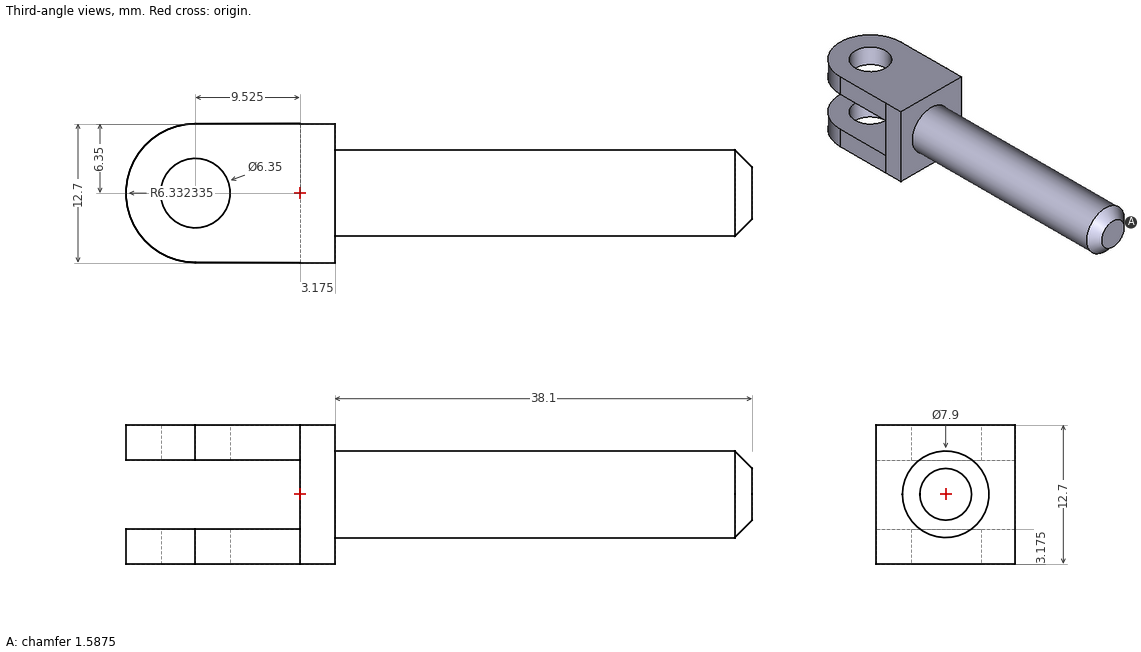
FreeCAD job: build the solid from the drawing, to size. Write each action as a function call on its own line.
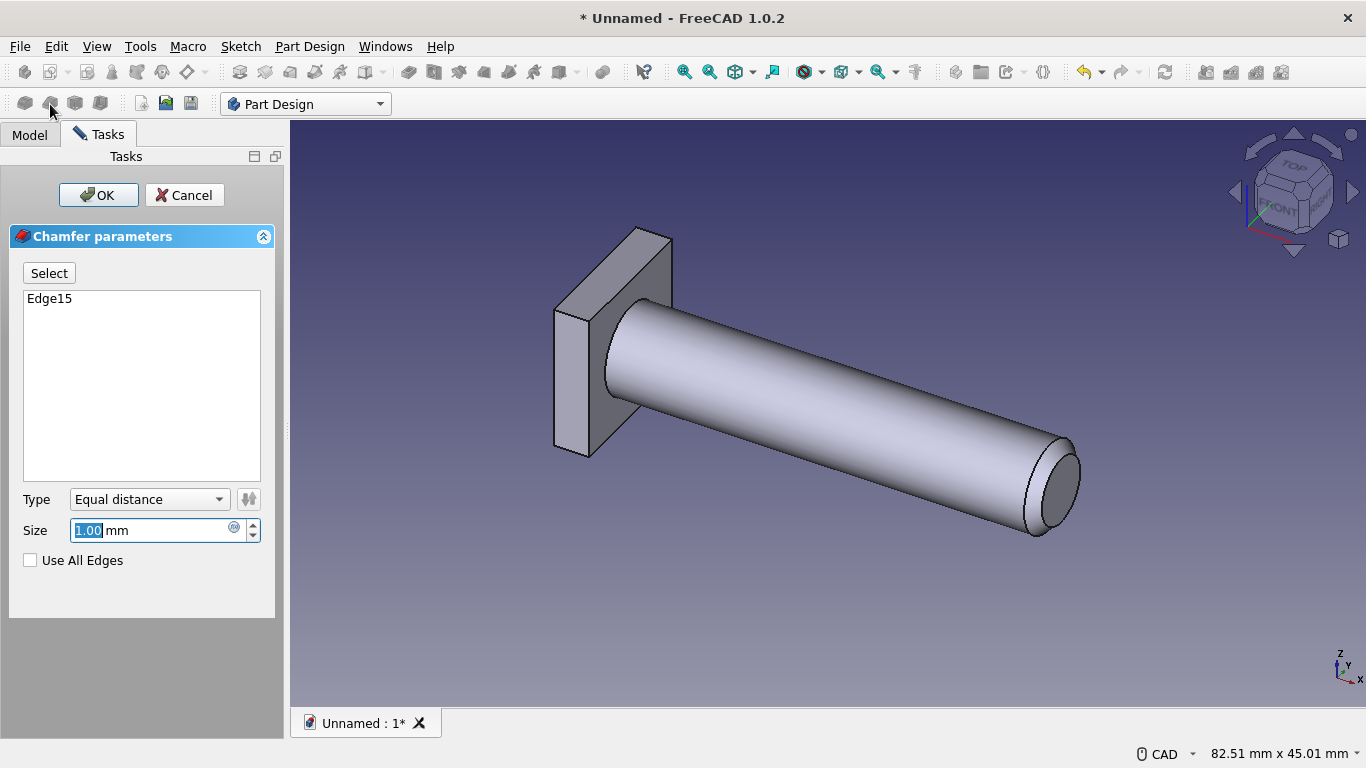
text(1.5875)
key(Tab)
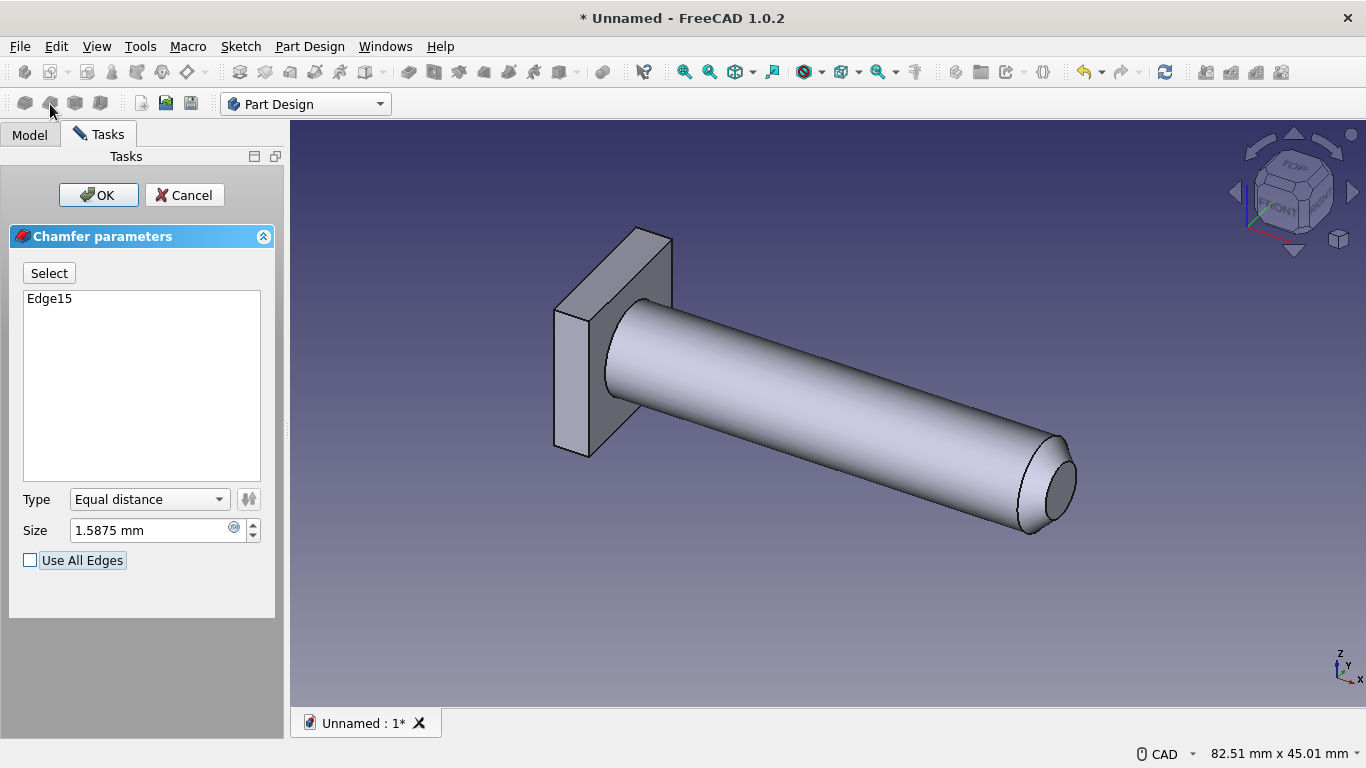
click(99, 195)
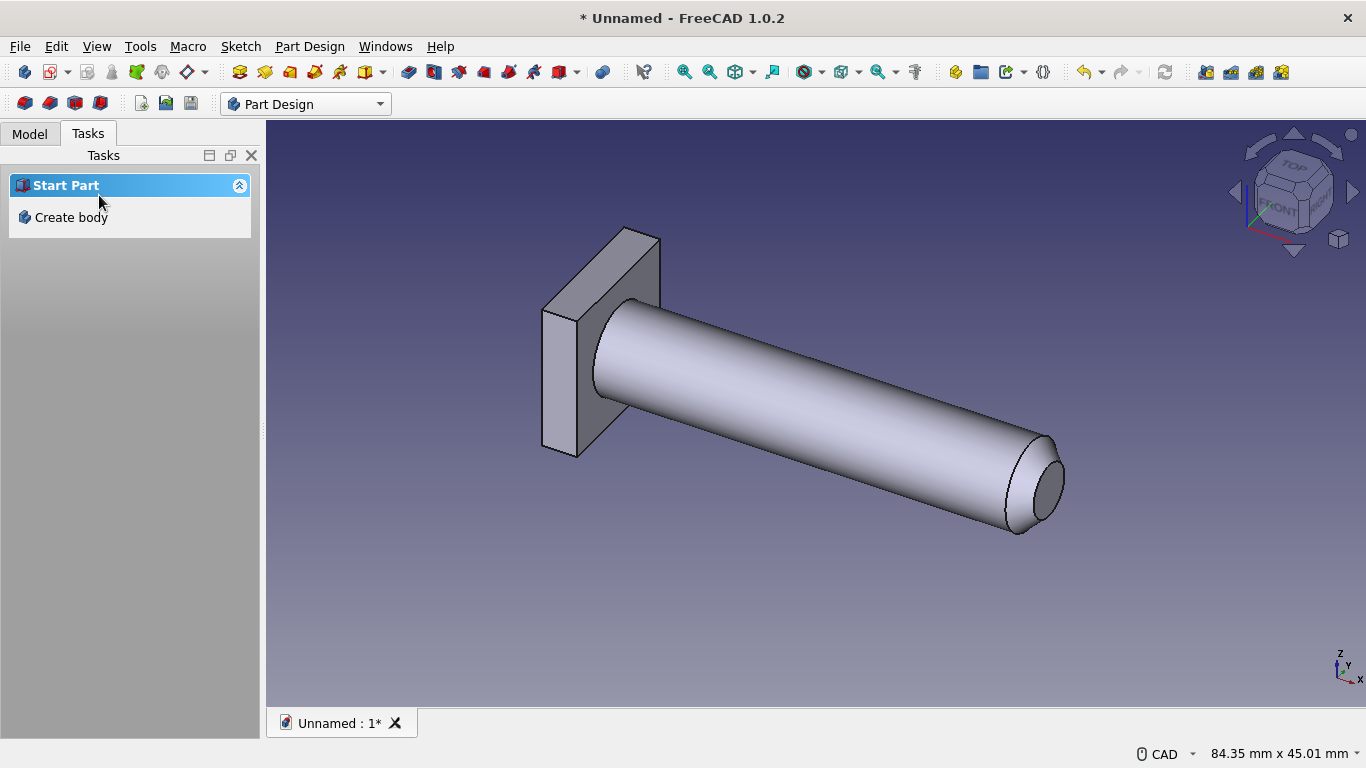
key(5)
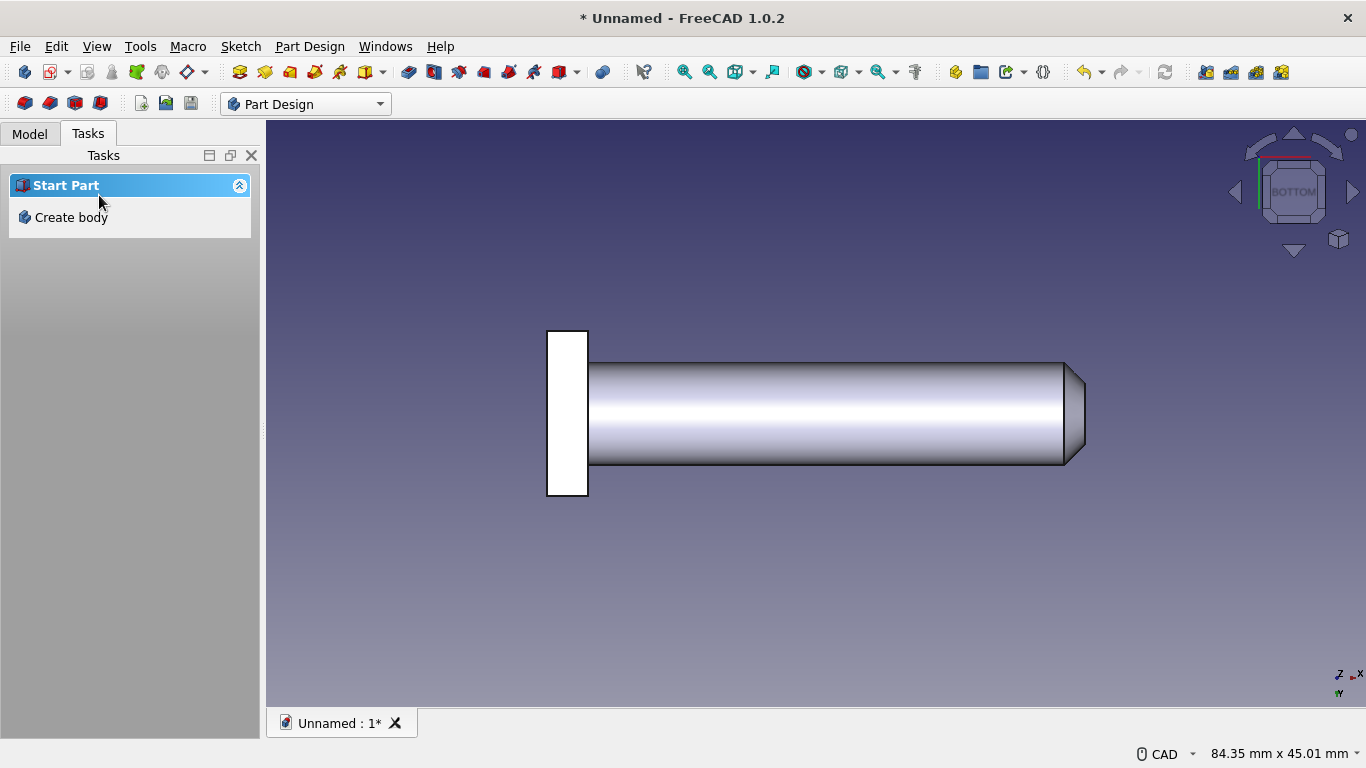
click(568, 460)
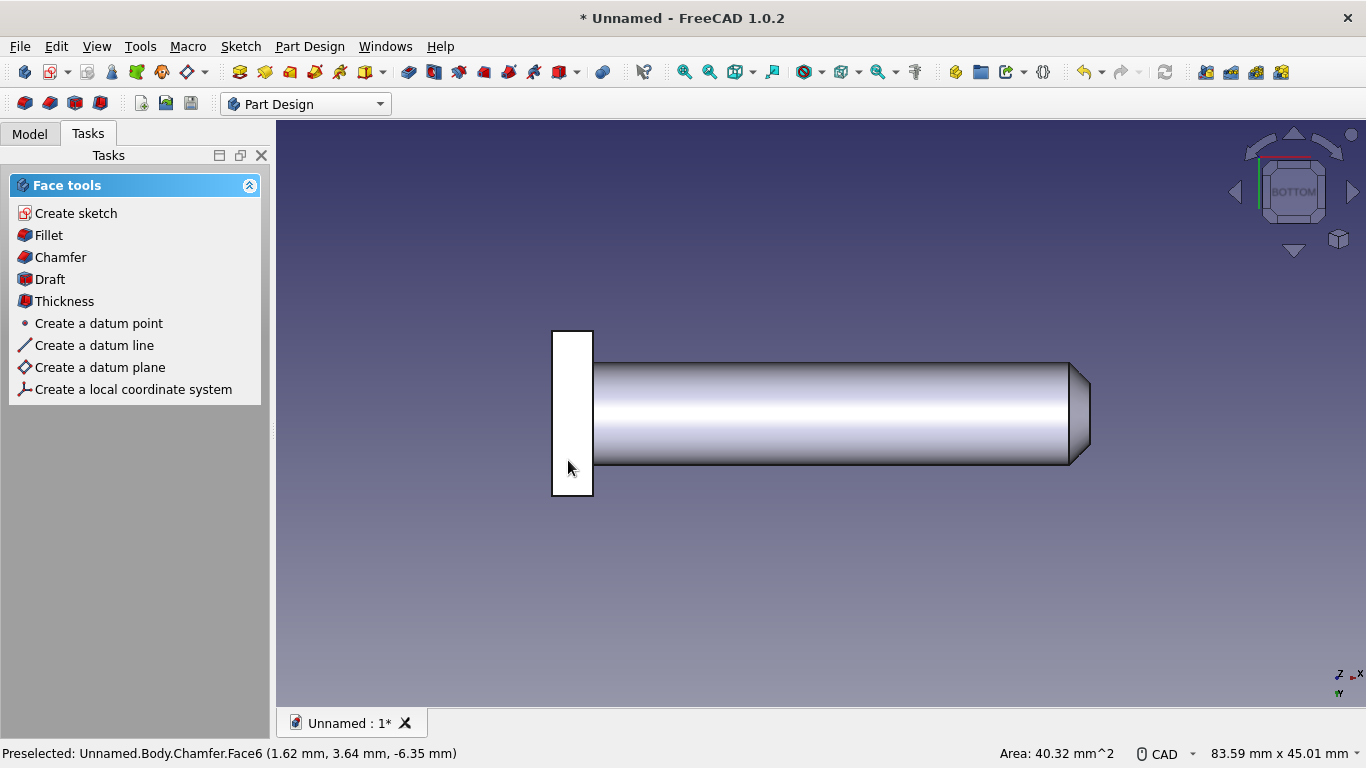
click(50, 72)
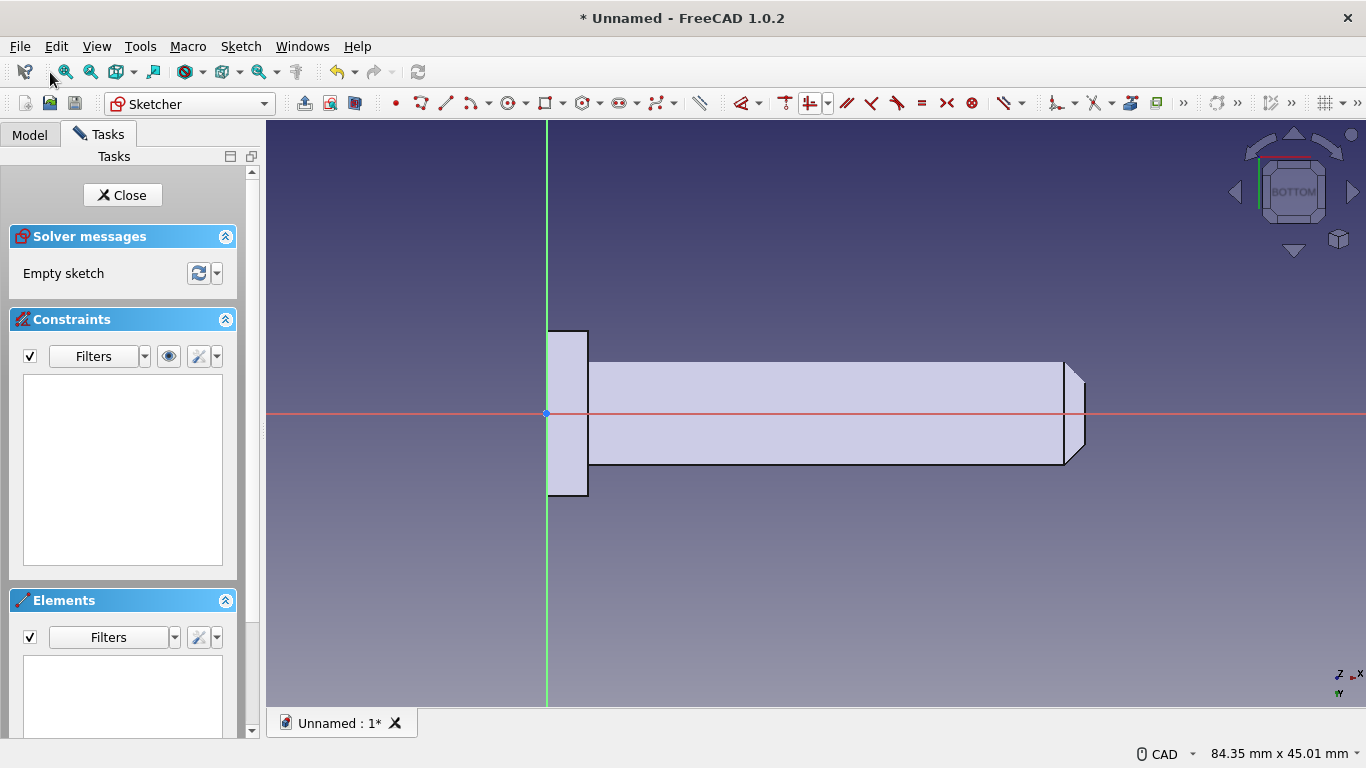
scroll(294, 413, up, 4)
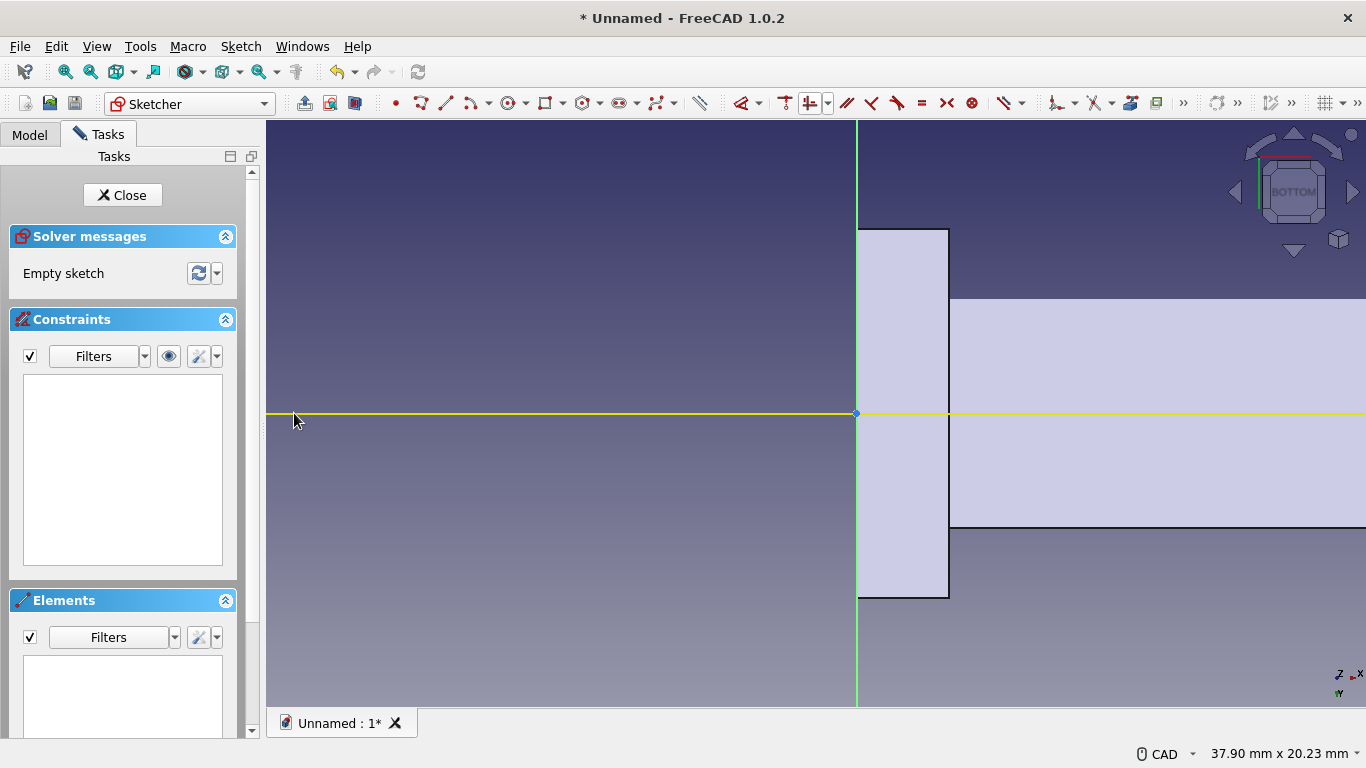
click(421, 104)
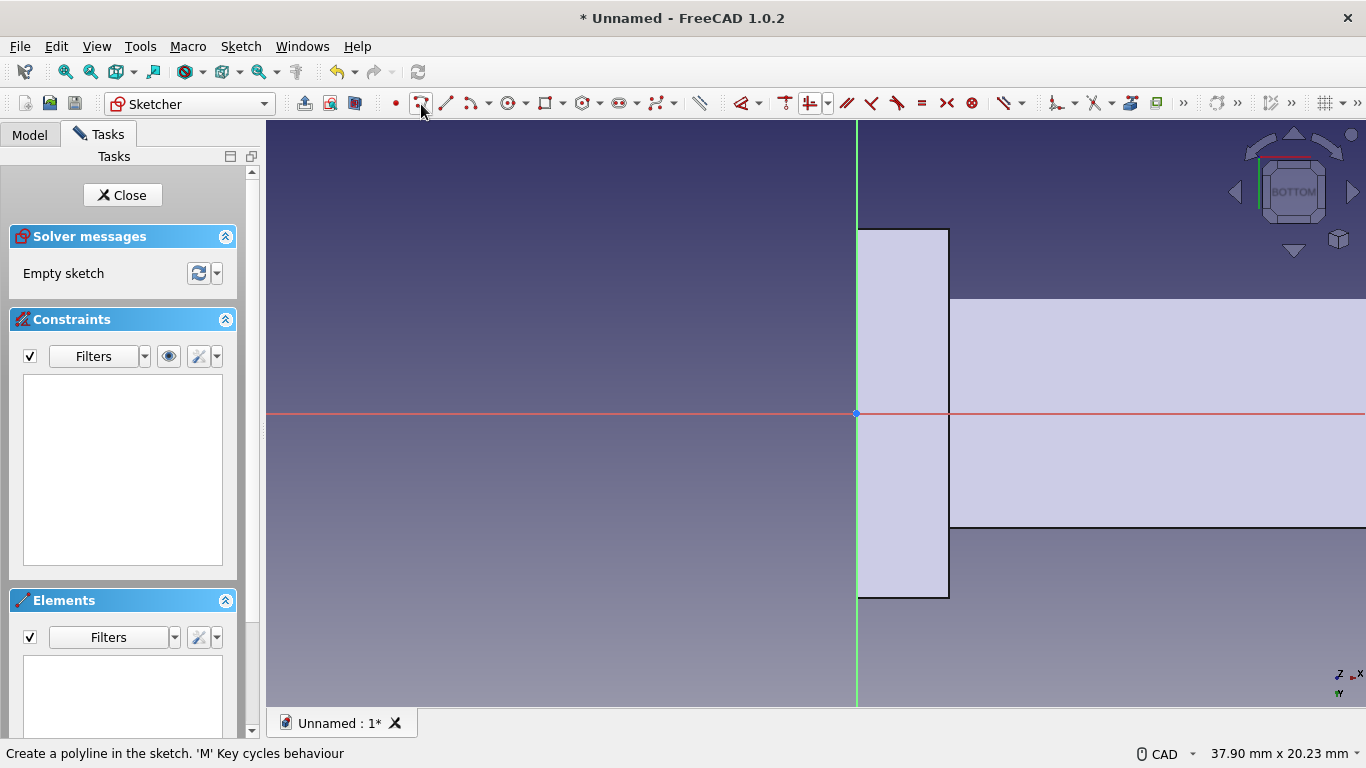
click(580, 597)
click(857, 611)
click(848, 229)
click(580, 243)
right_click(580, 243)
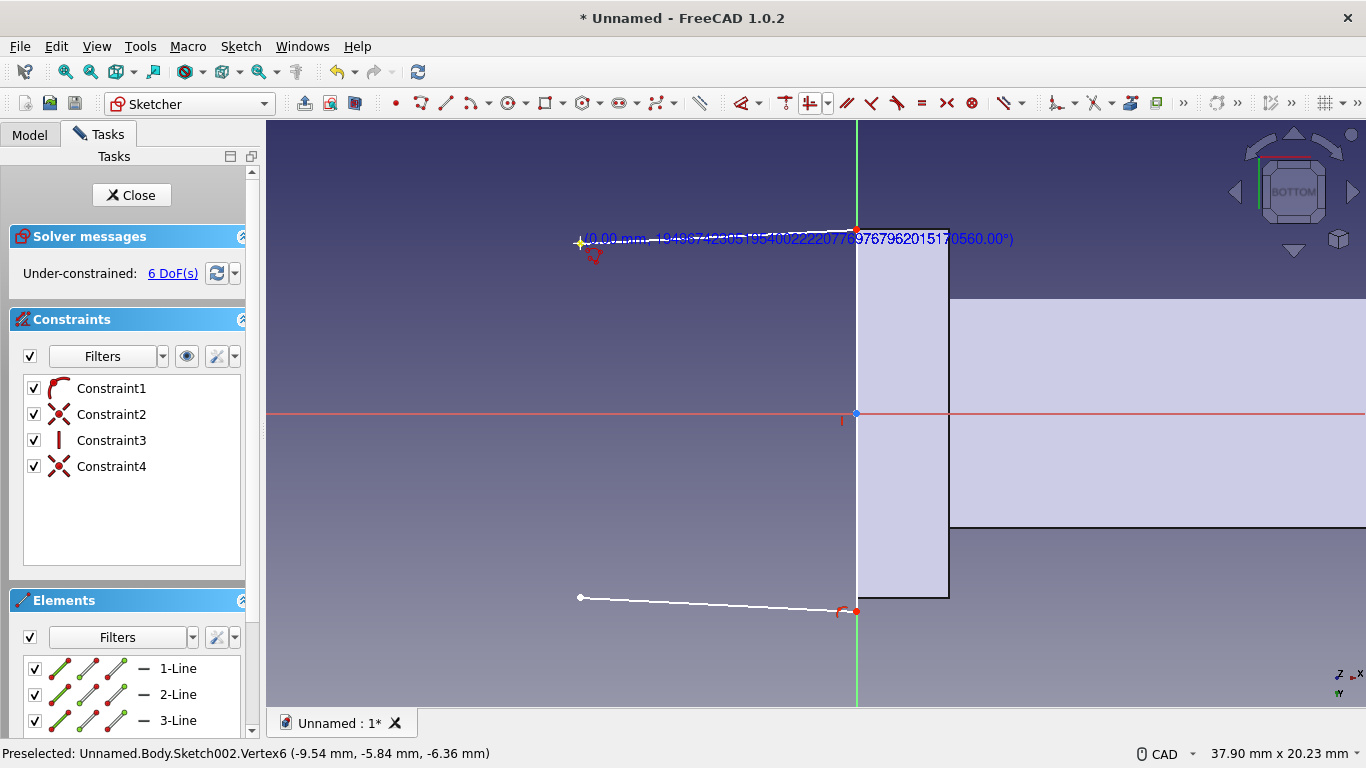
key(g)
key(3)
key(a)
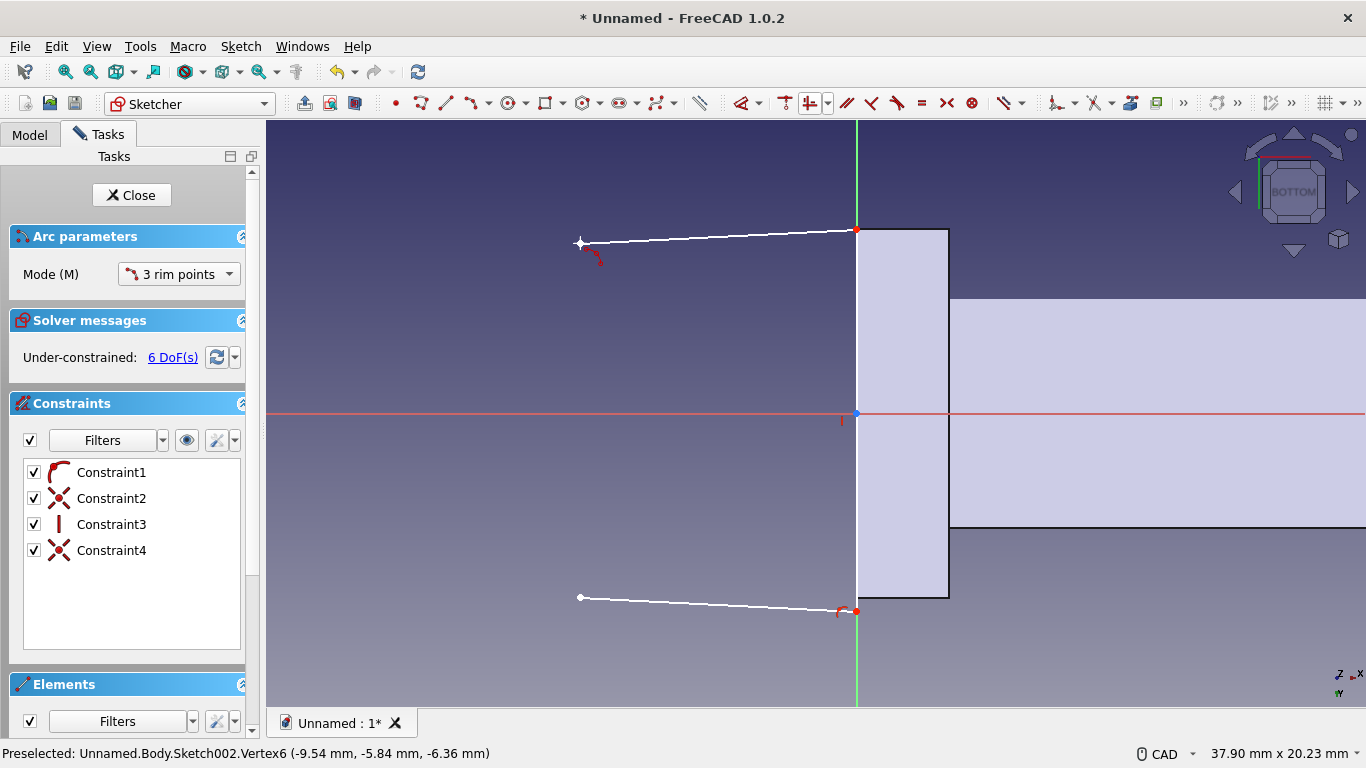
click(580, 244)
click(580, 598)
click(406, 357)